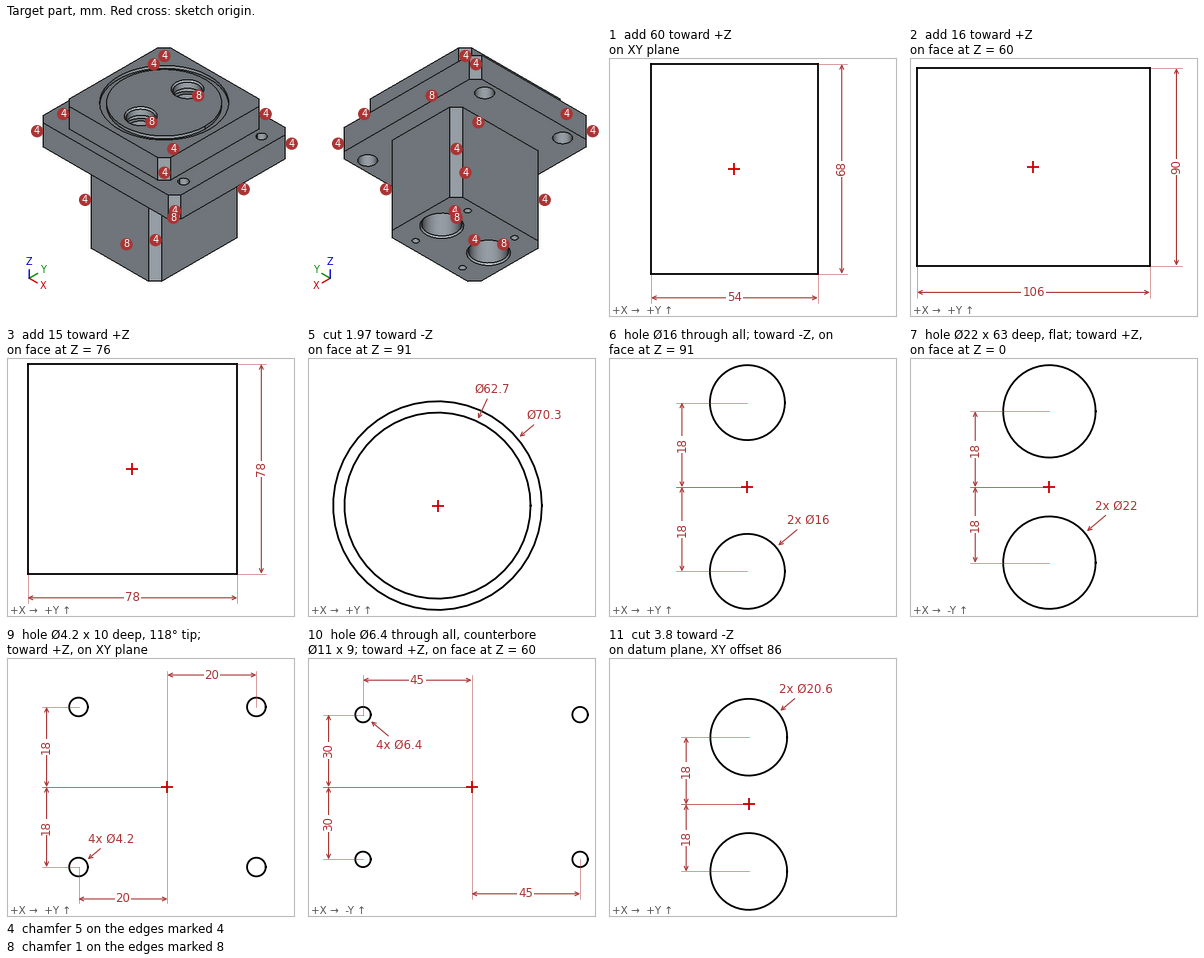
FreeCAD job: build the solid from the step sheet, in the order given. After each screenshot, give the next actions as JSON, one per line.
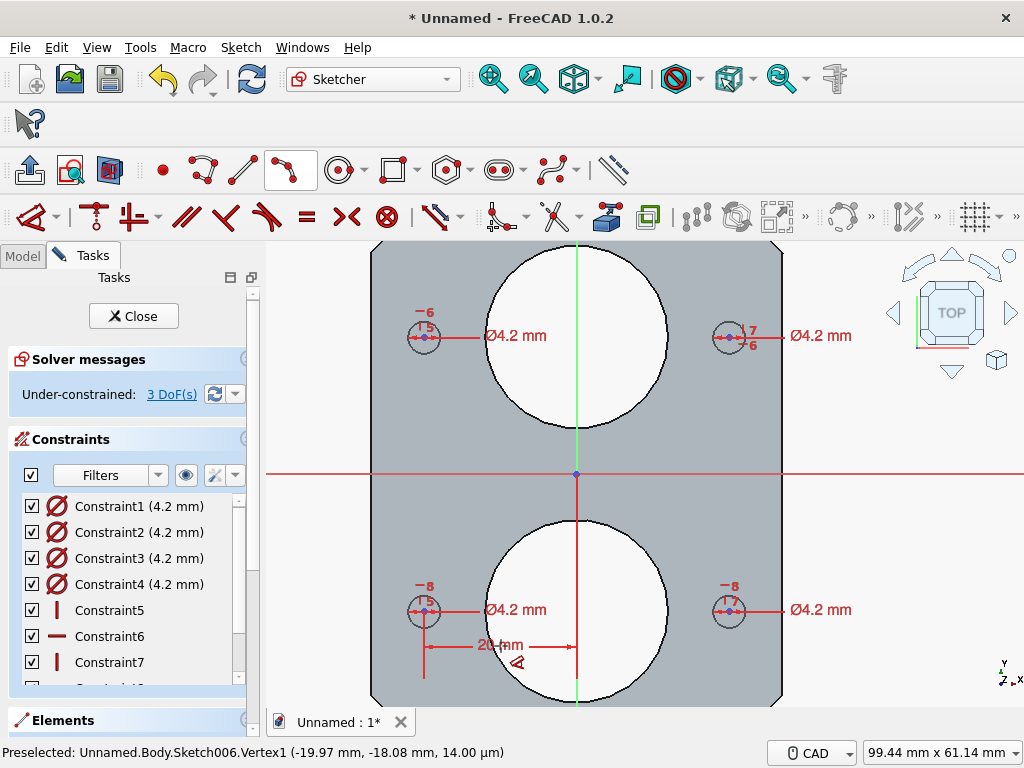
{"action": "left_click", "coordinate": [424, 612]}
{"action": "left_click", "coordinate": [390, 543]}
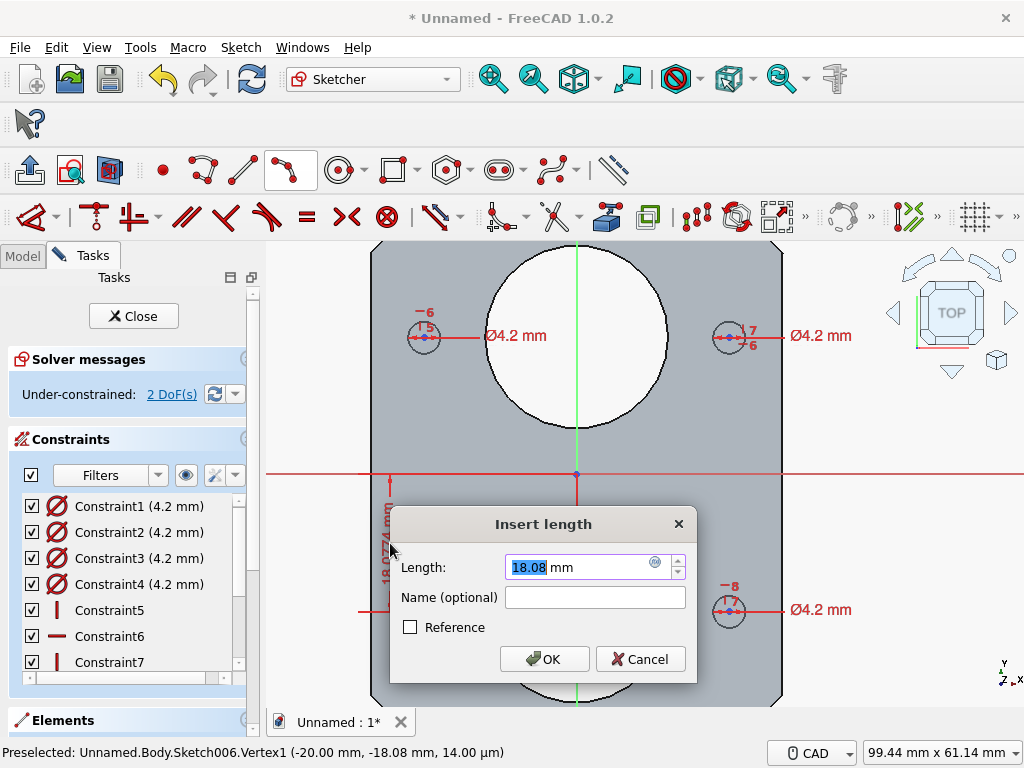
{"action": "type", "text": "18"}
{"action": "key", "text": "Return"}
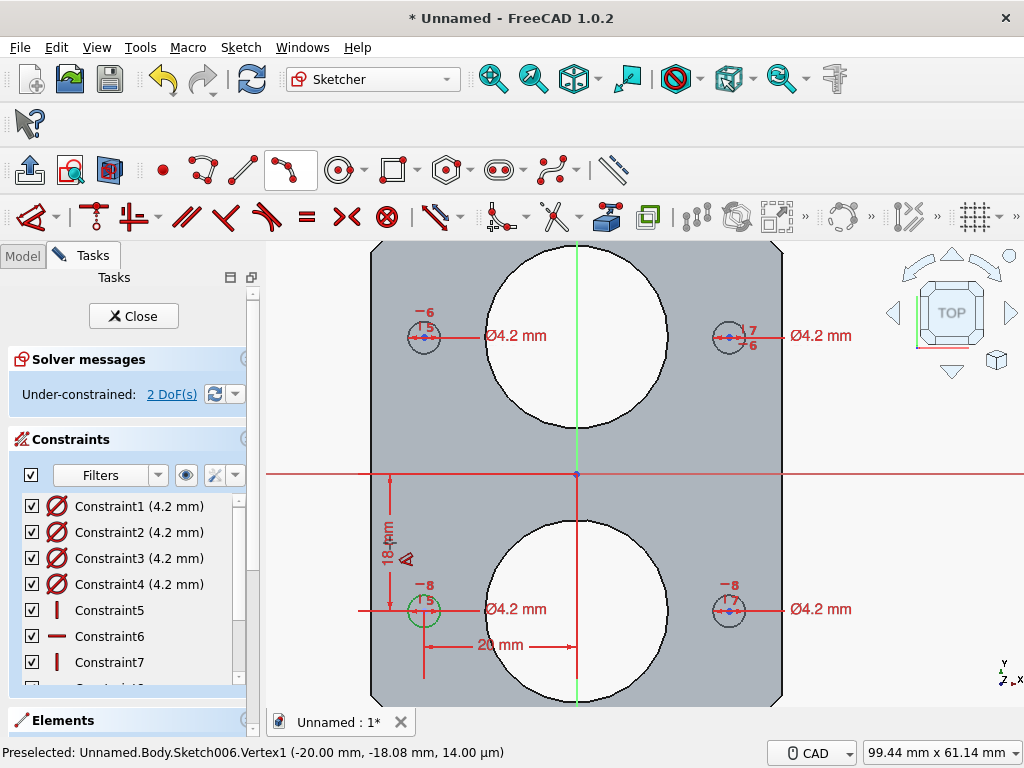
{"action": "left_click", "coordinate": [424, 338]}
{"action": "left_click", "coordinate": [390, 406]}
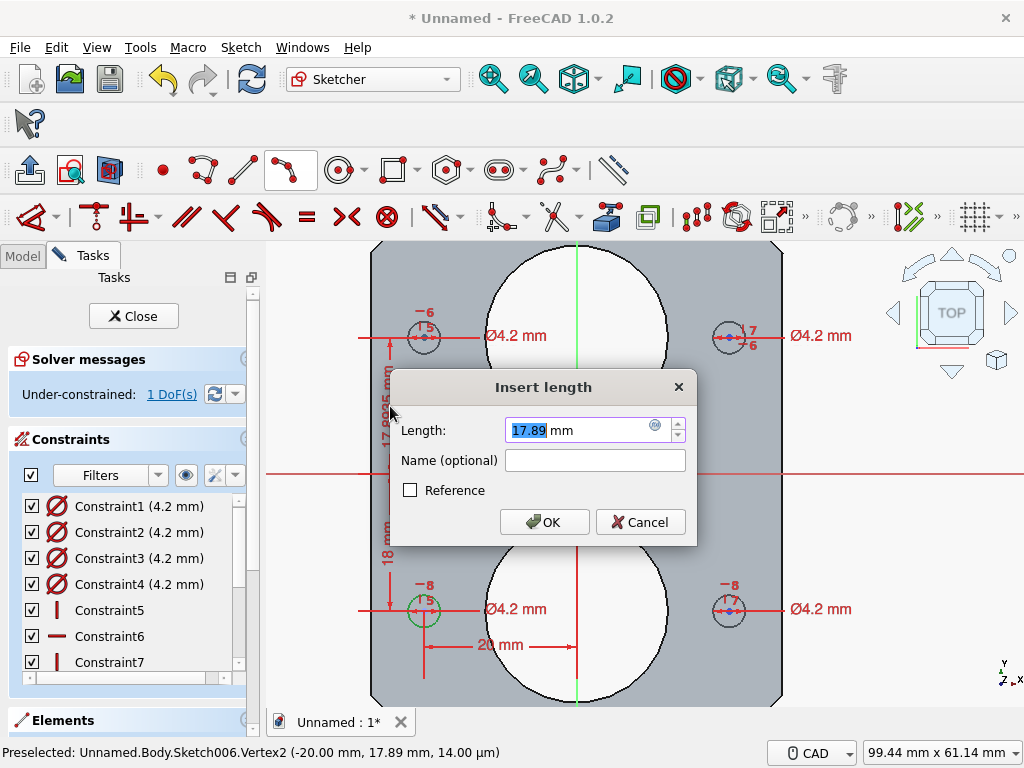
{"action": "type", "text": "18"}
{"action": "key", "text": "Return"}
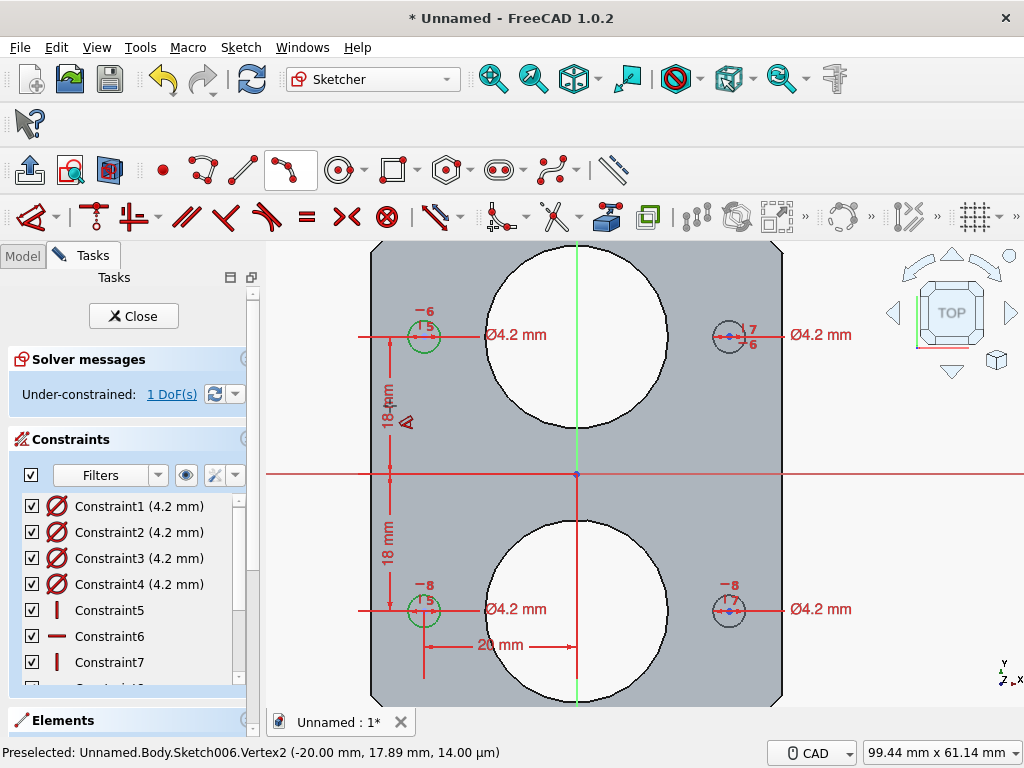
{"action": "left_click", "coordinate": [729, 337]}
{"action": "left_click", "coordinate": [653, 303]}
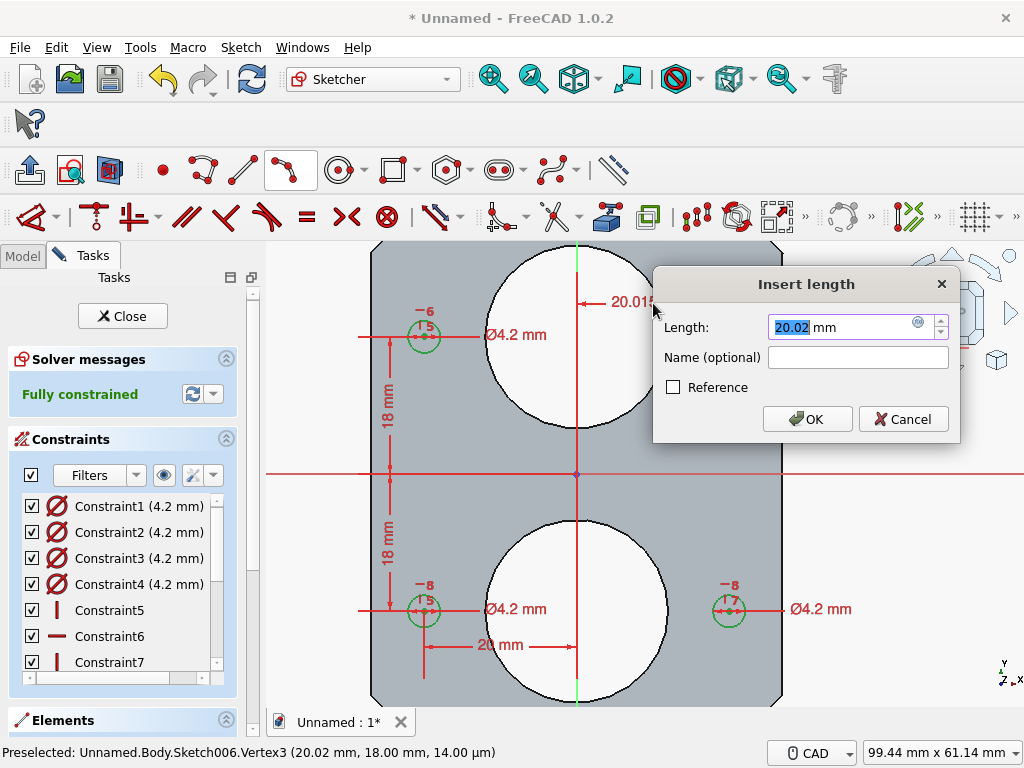
{"action": "type", "text": "20"}
{"action": "key", "text": "Return"}
{"action": "key", "text": "Escape"}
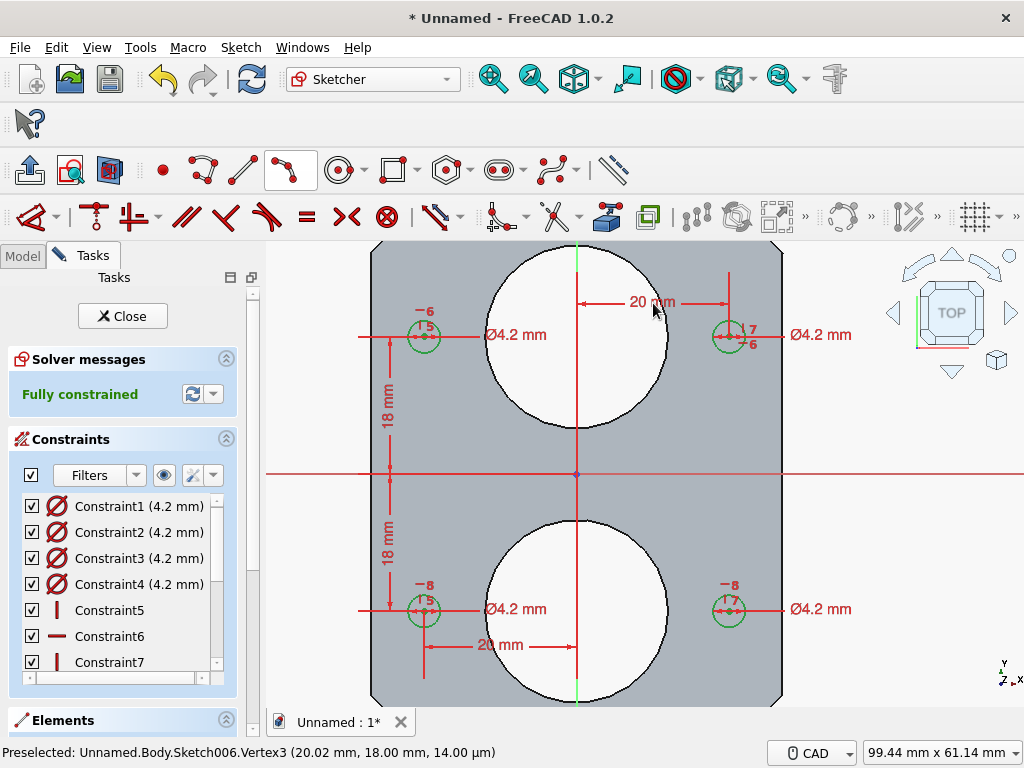
{"action": "left_click", "coordinate": [123, 316]}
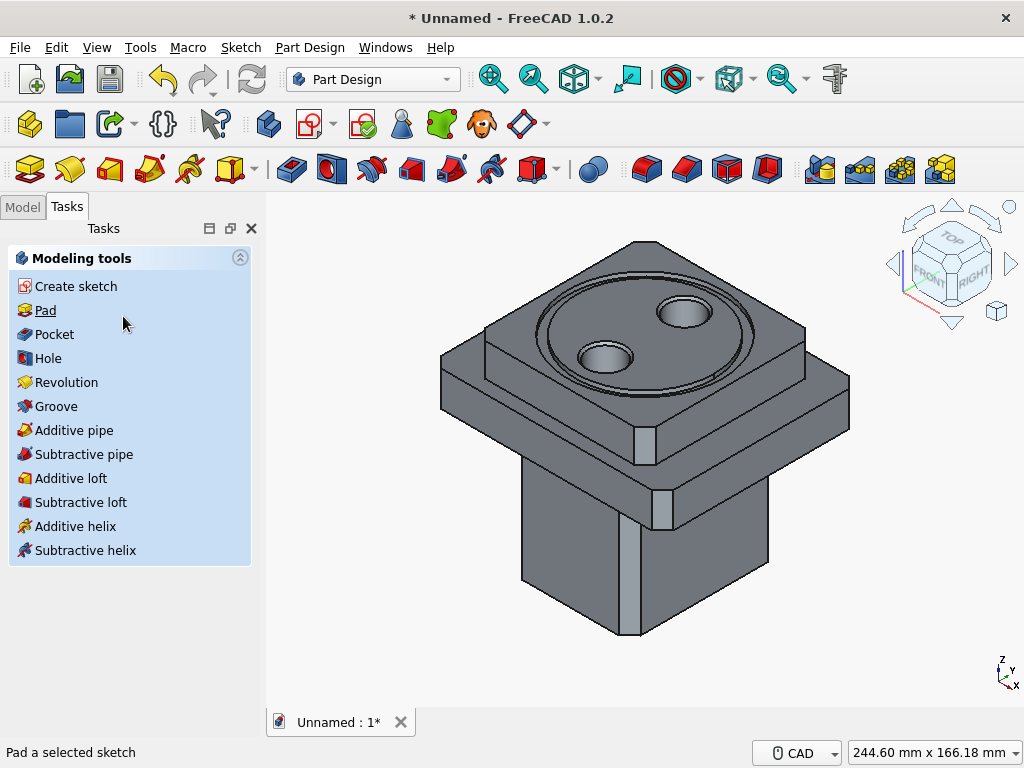
{"action": "left_click", "coordinate": [332, 170]}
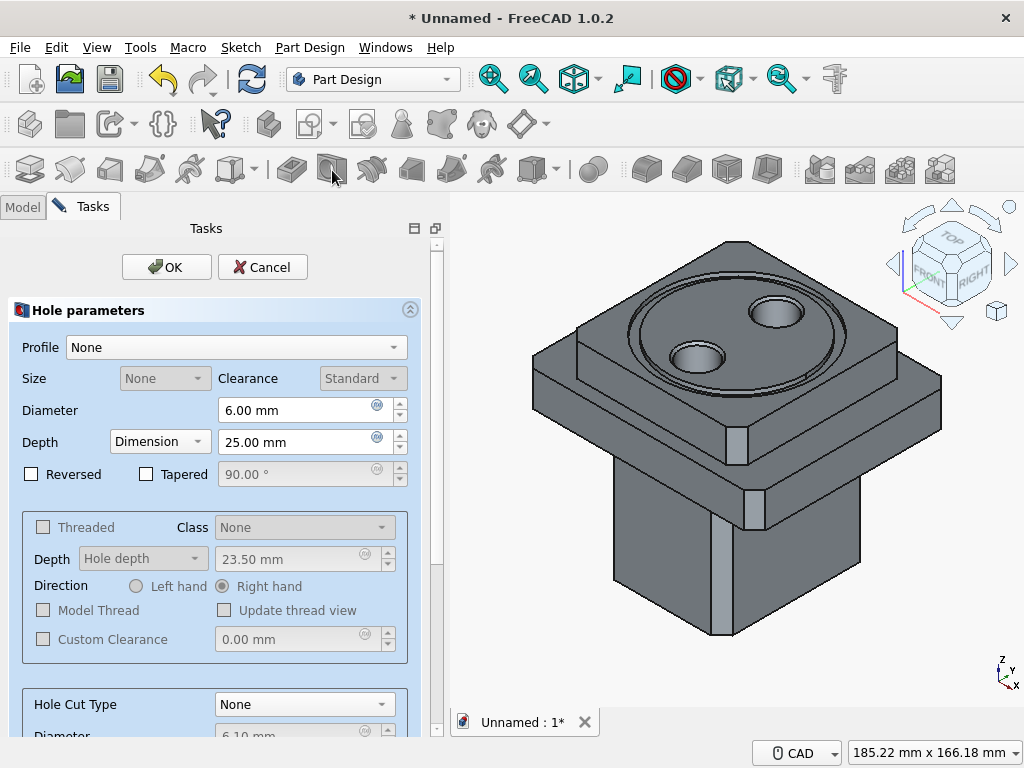
{"action": "triple_click", "coordinate": [305, 410]}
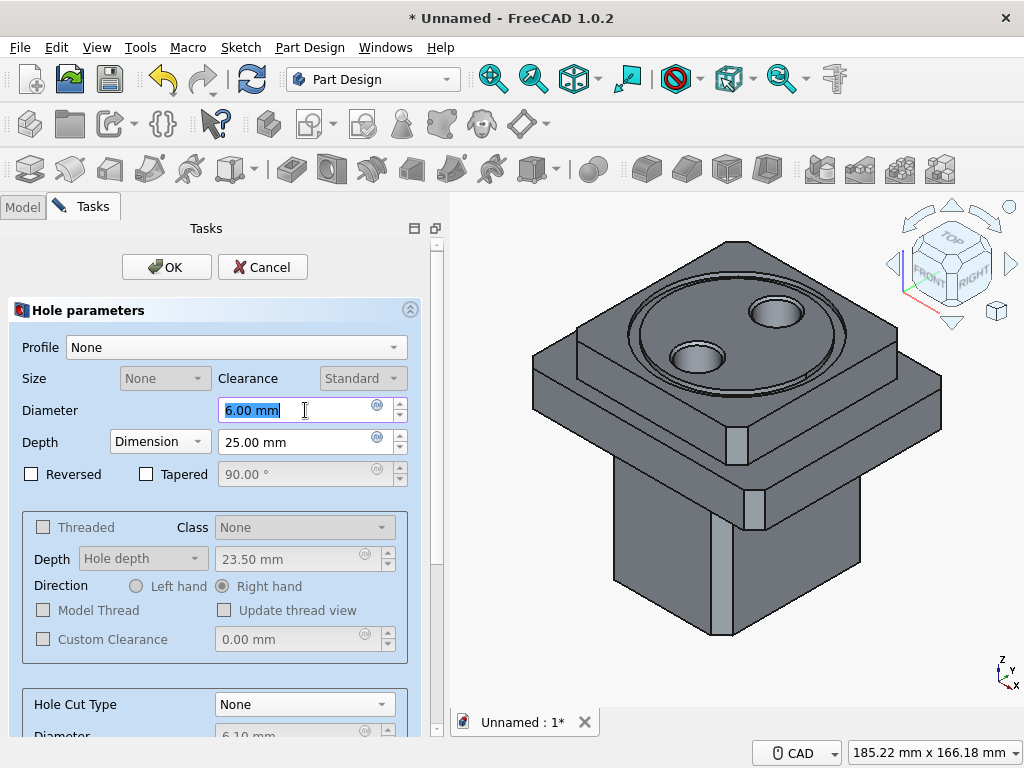
{"action": "type", "text": "4.2"}
{"action": "key", "text": "Tab"}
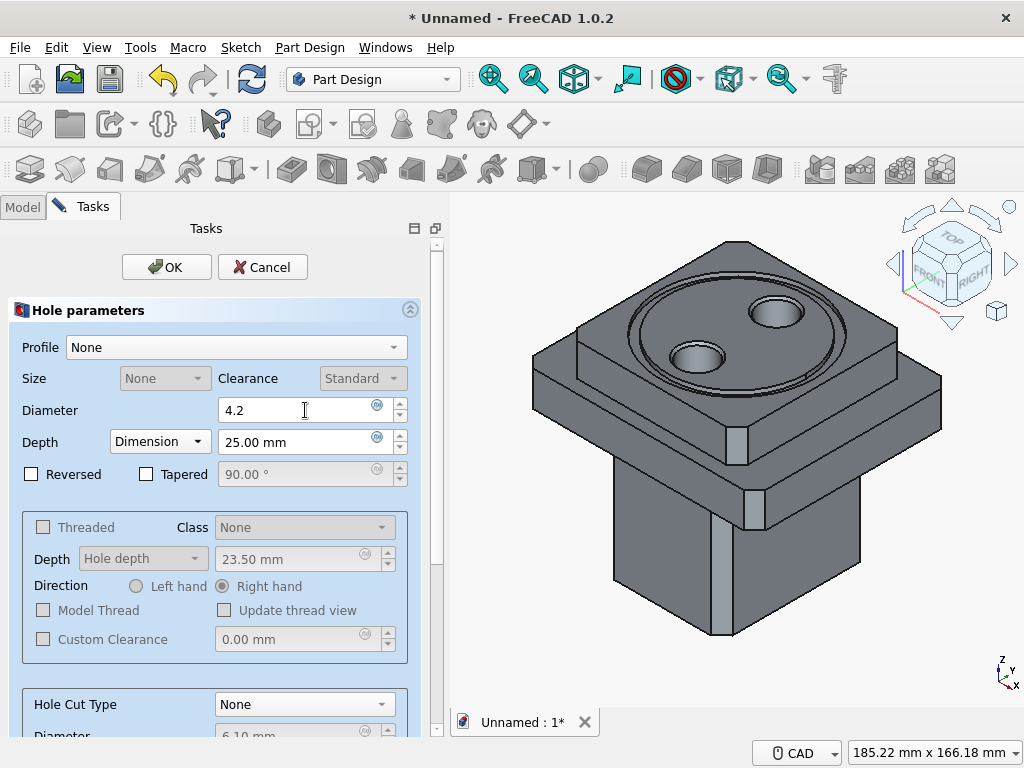
{"action": "triple_click", "coordinate": [305, 442]}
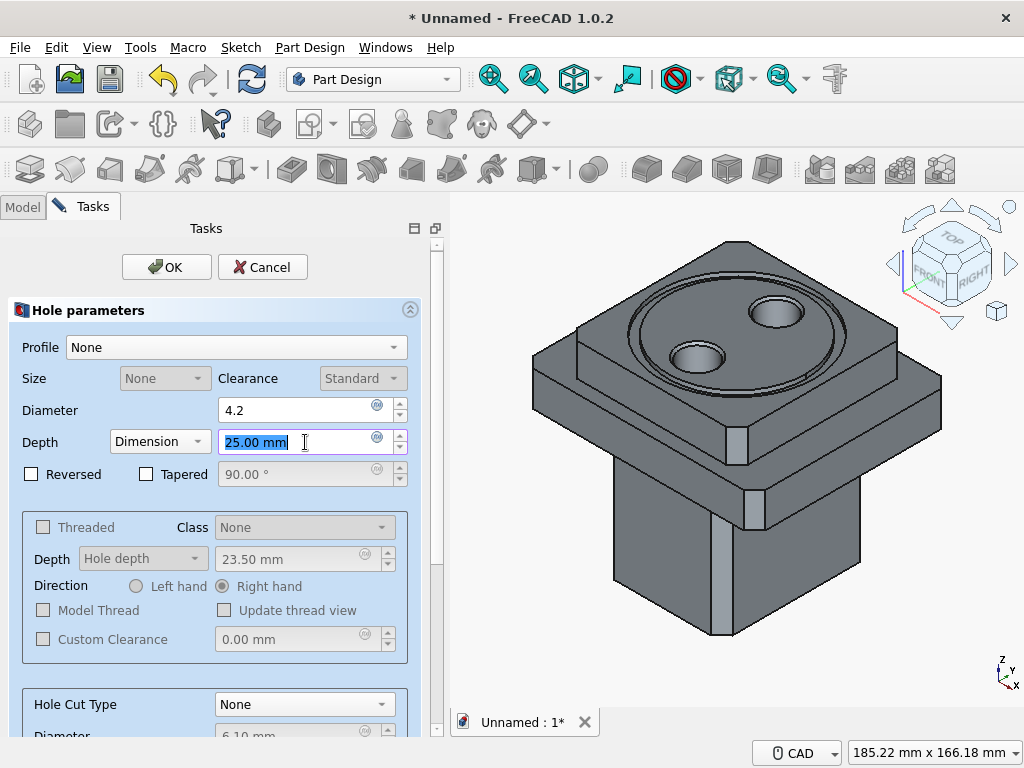
{"action": "type", "text": "10"}
{"action": "key", "text": "Tab"}